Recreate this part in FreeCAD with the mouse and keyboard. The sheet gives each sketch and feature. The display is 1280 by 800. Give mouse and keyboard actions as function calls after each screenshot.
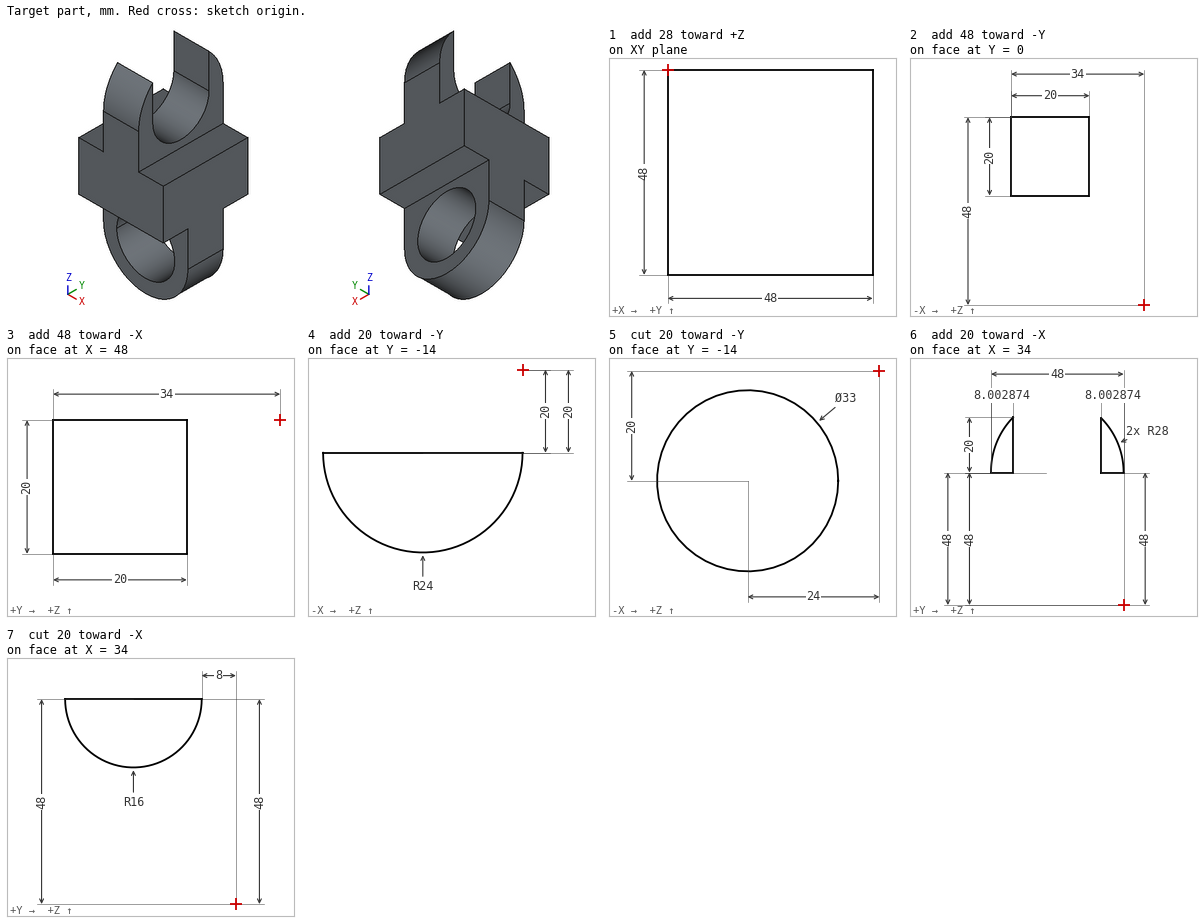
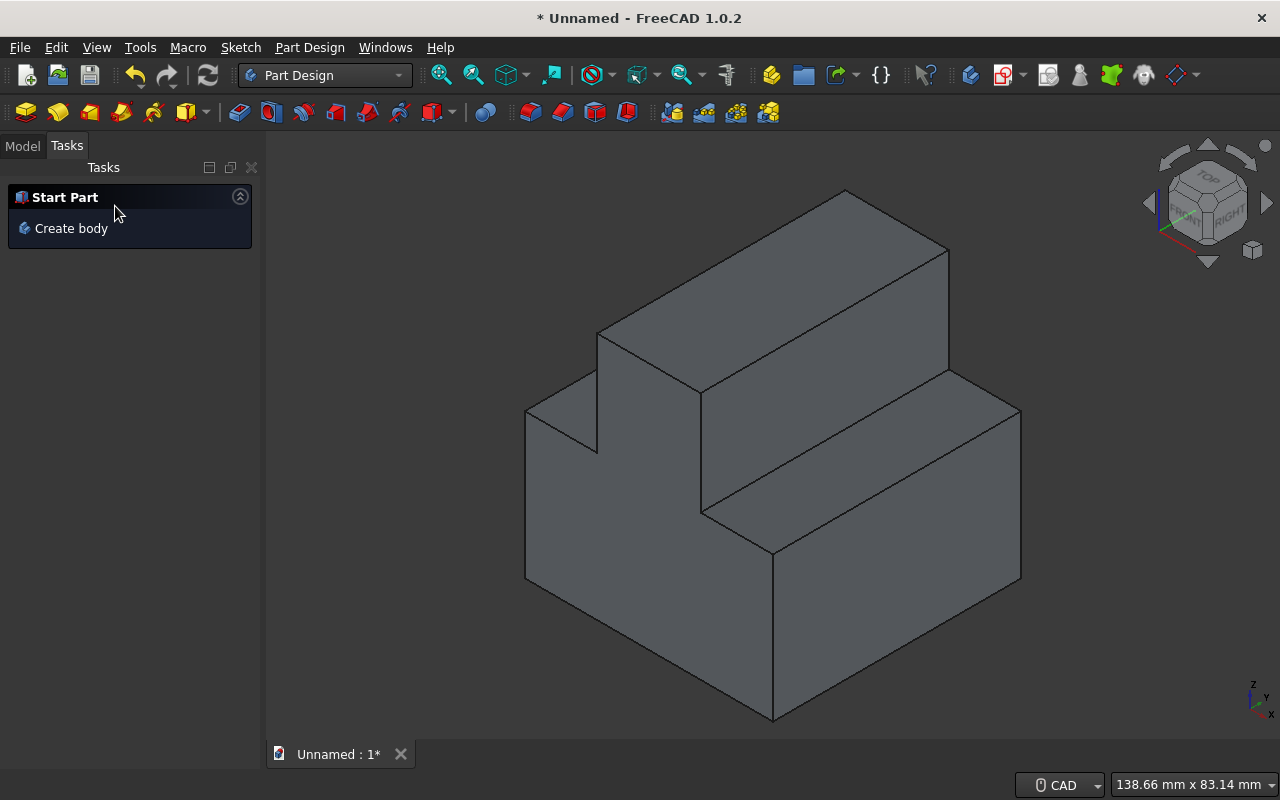
click(933, 545)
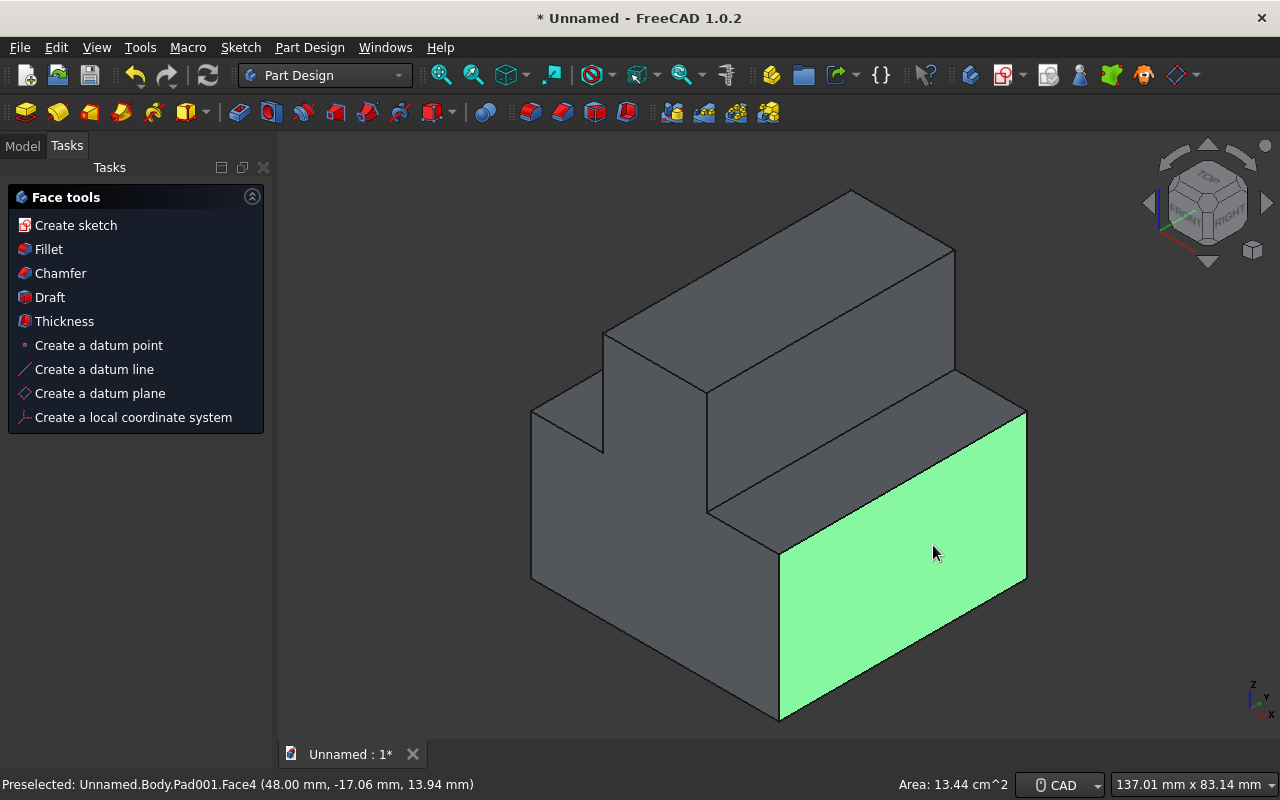
click(1004, 76)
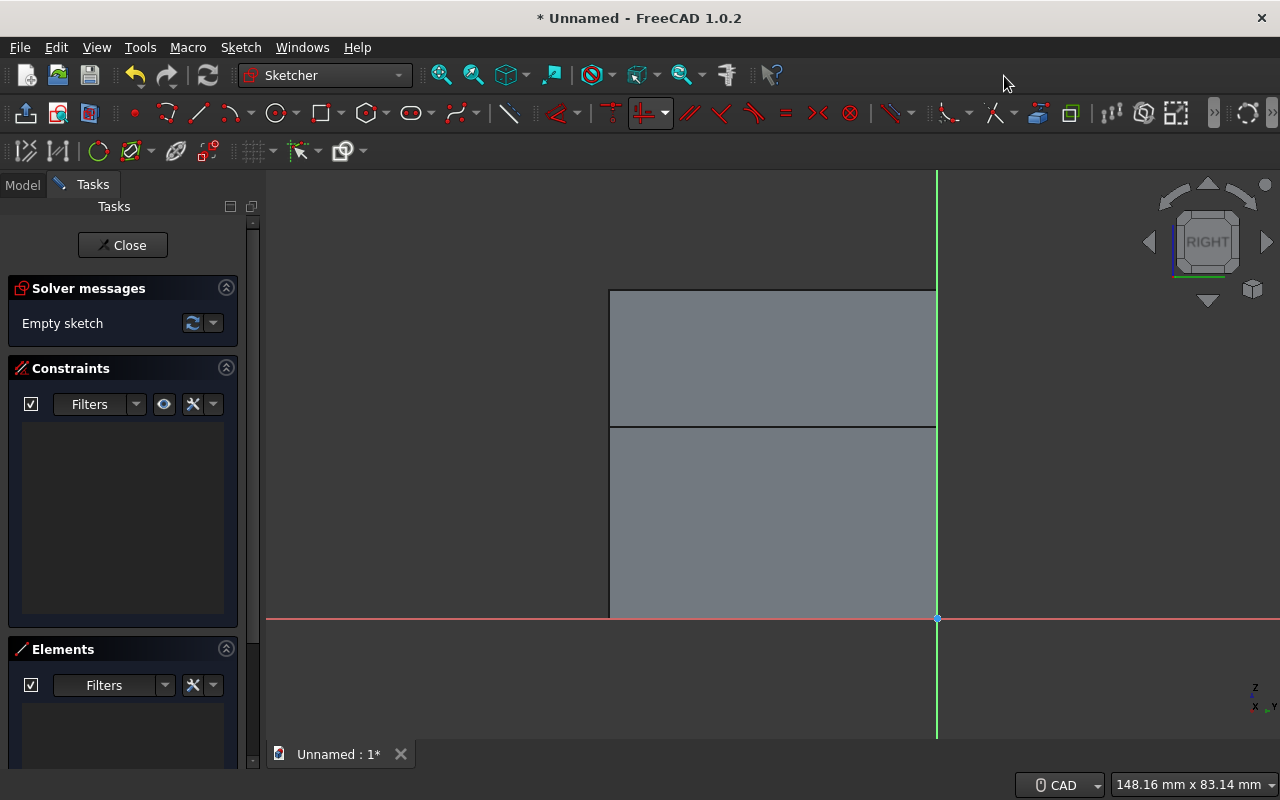
scroll(704, 454, down, 5)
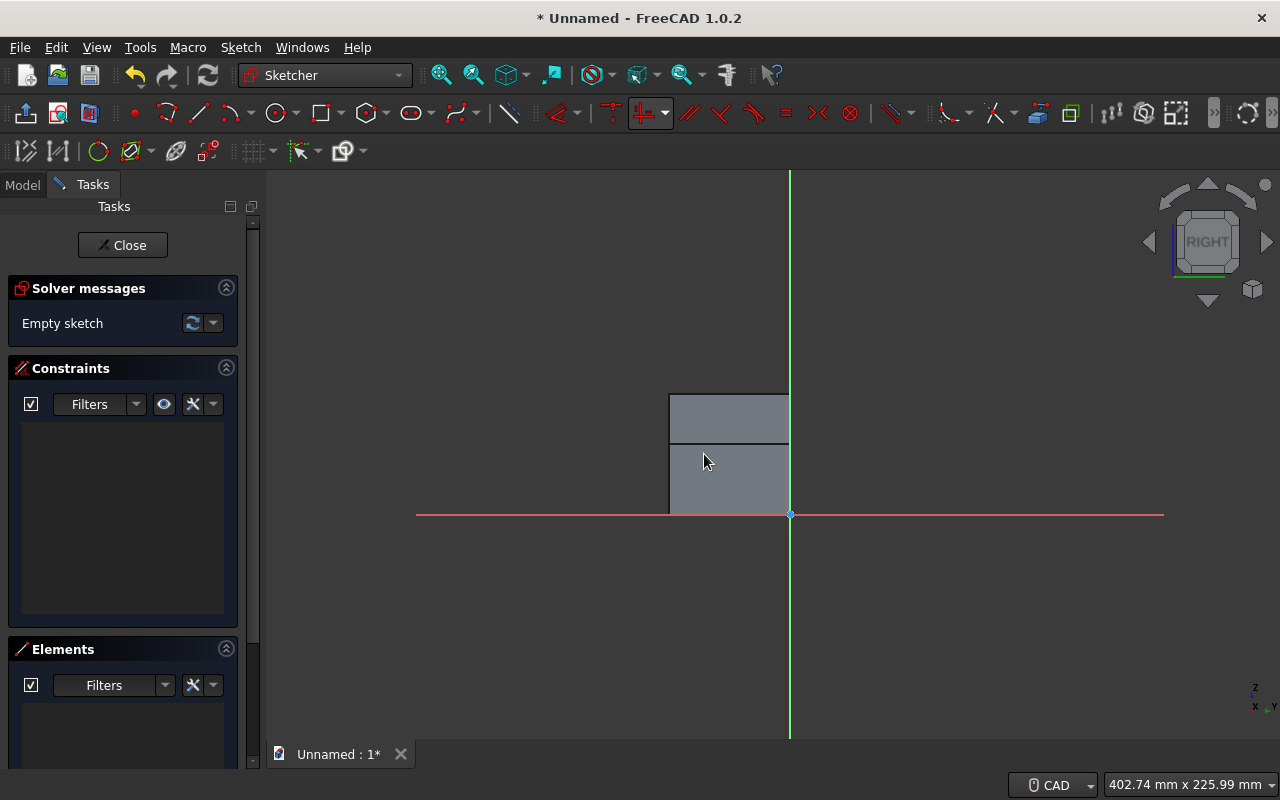
scroll(754, 554, up, 10)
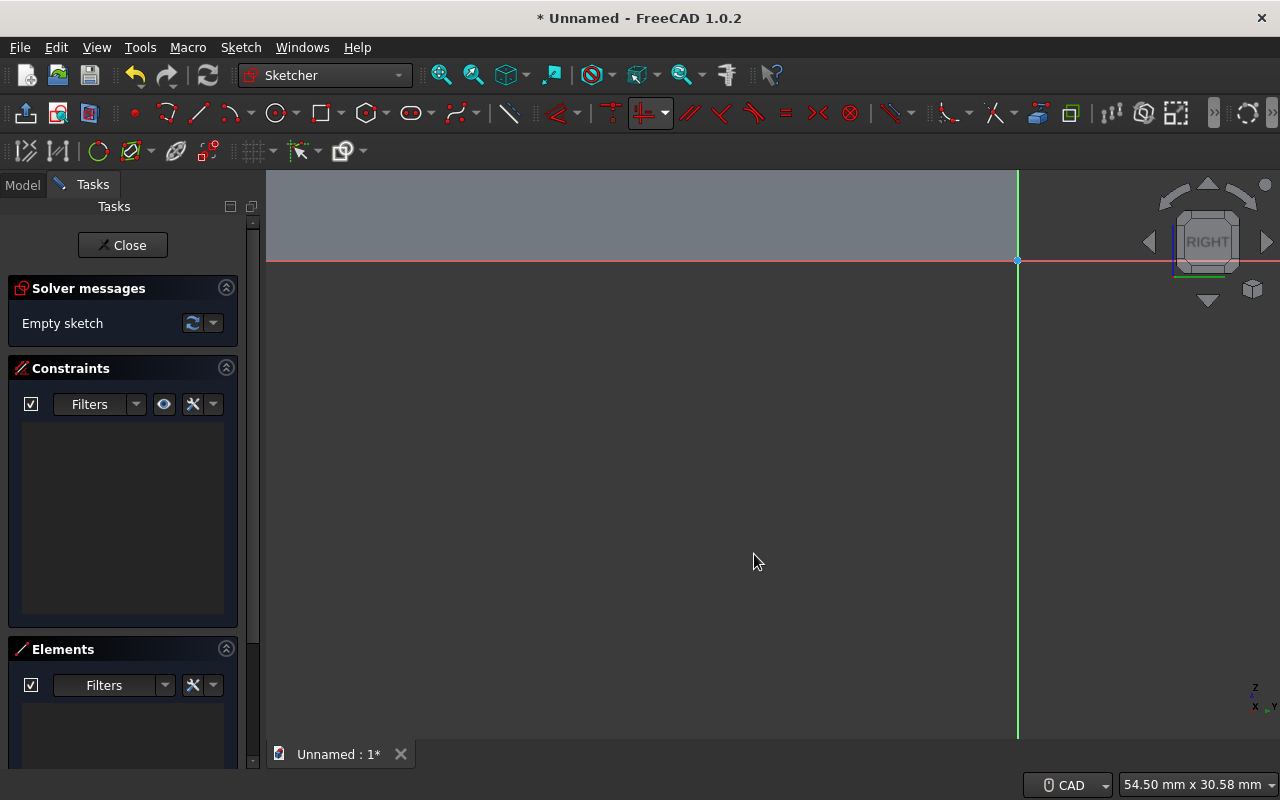
key(g)
key(r)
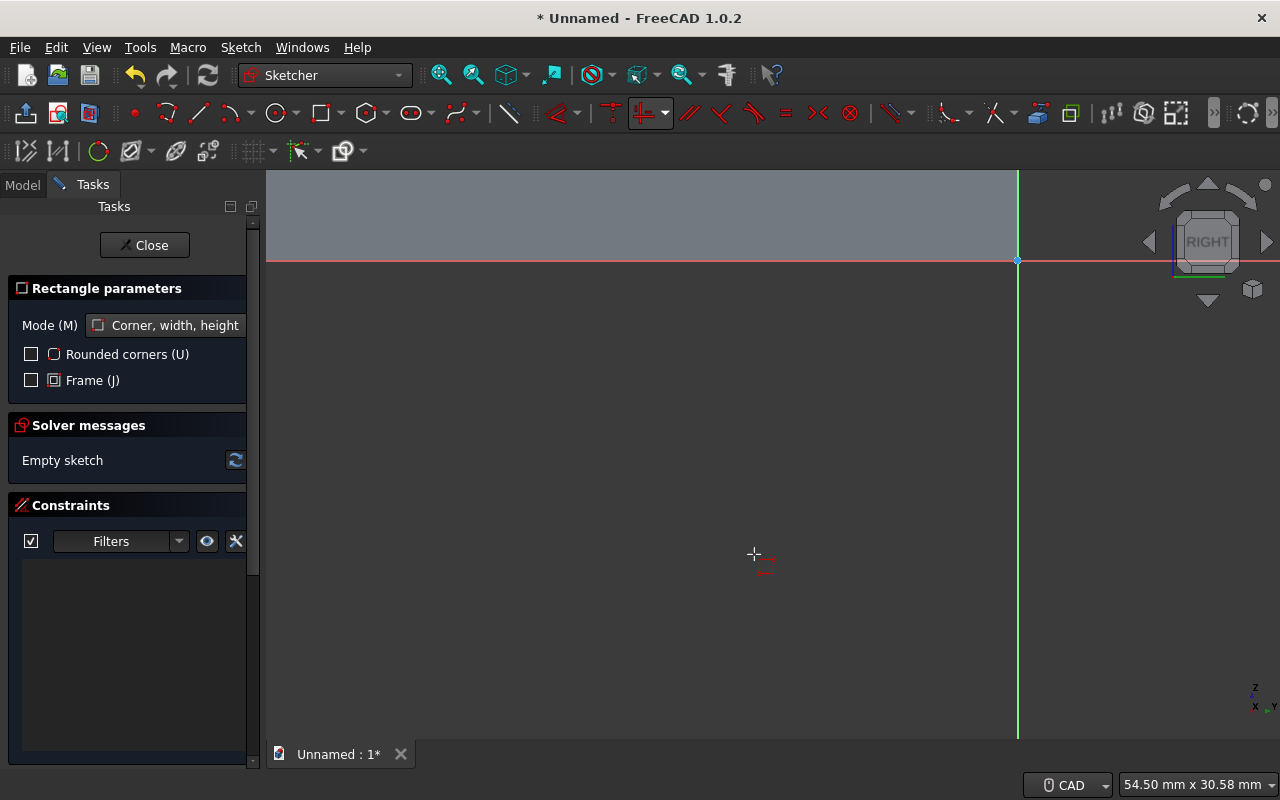
click(385, 261)
click(757, 633)
key(Escape)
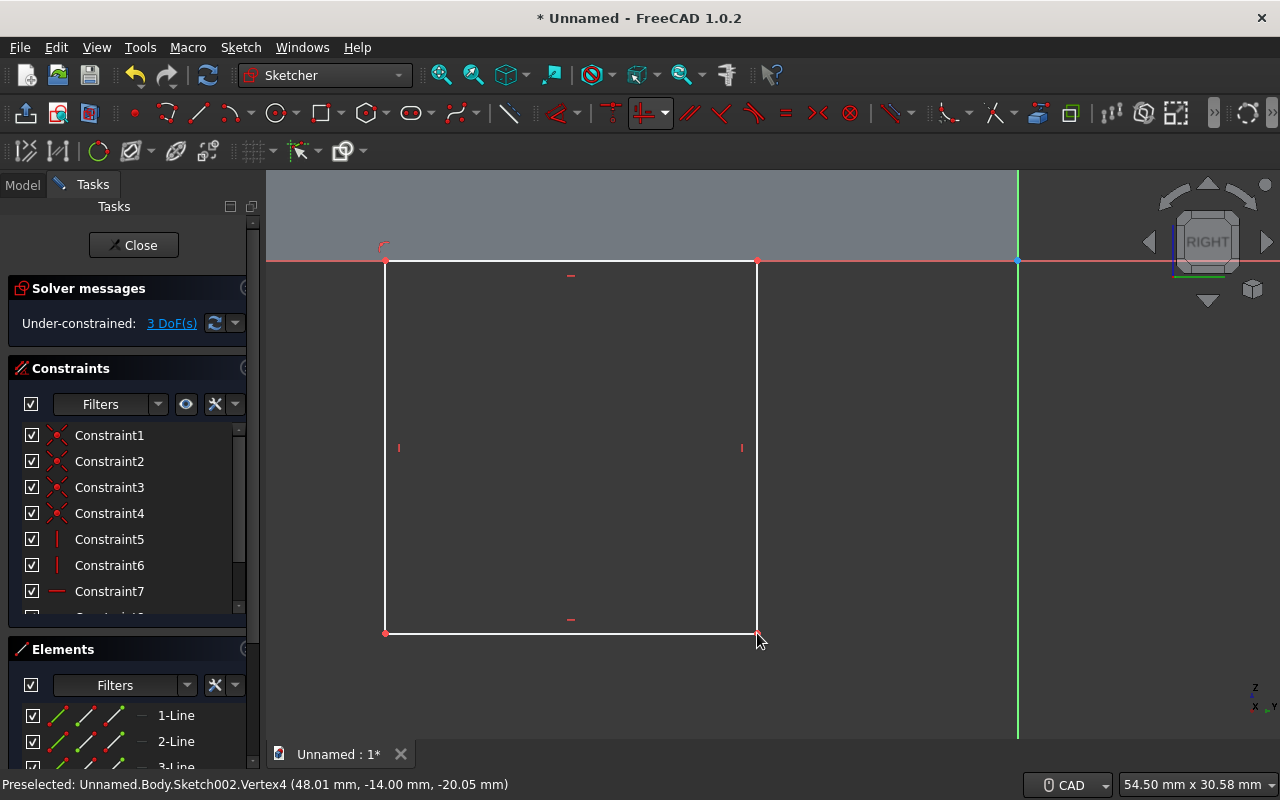
key(d)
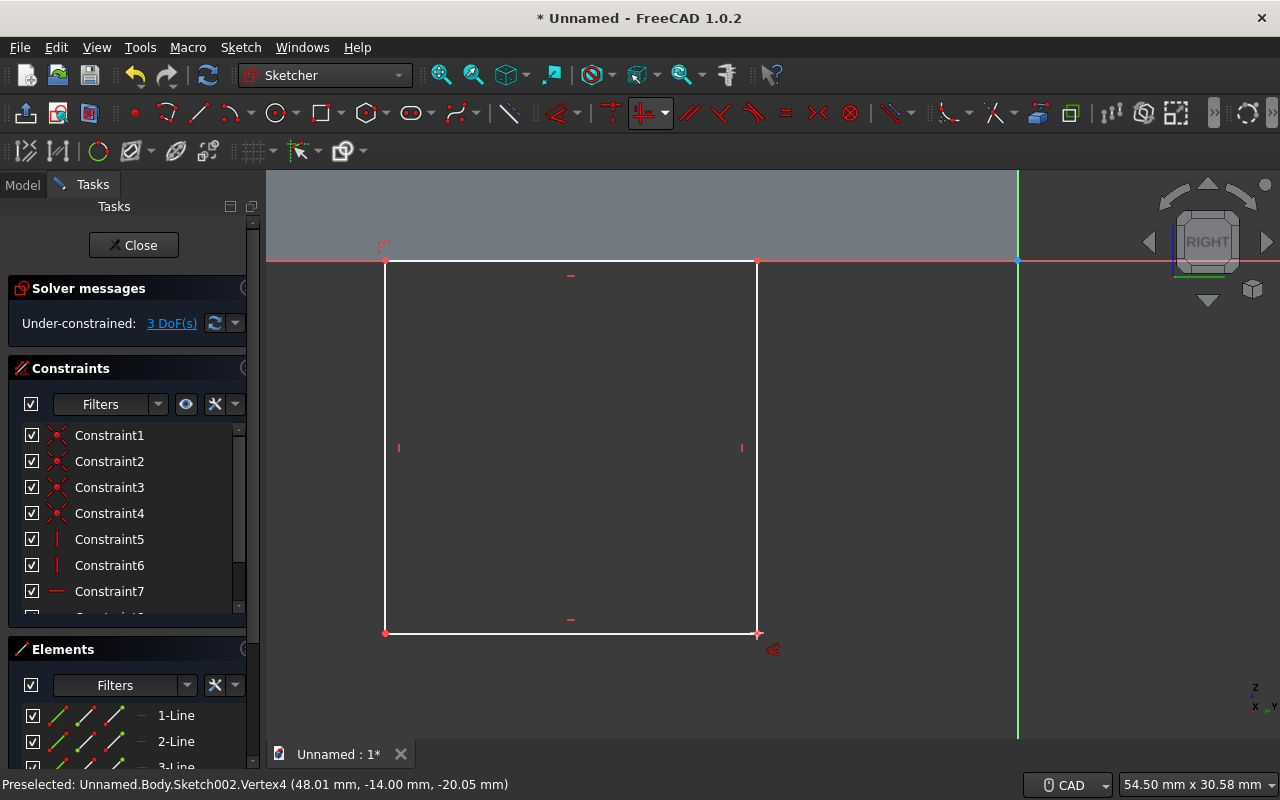
click(385, 373)
click(351, 447)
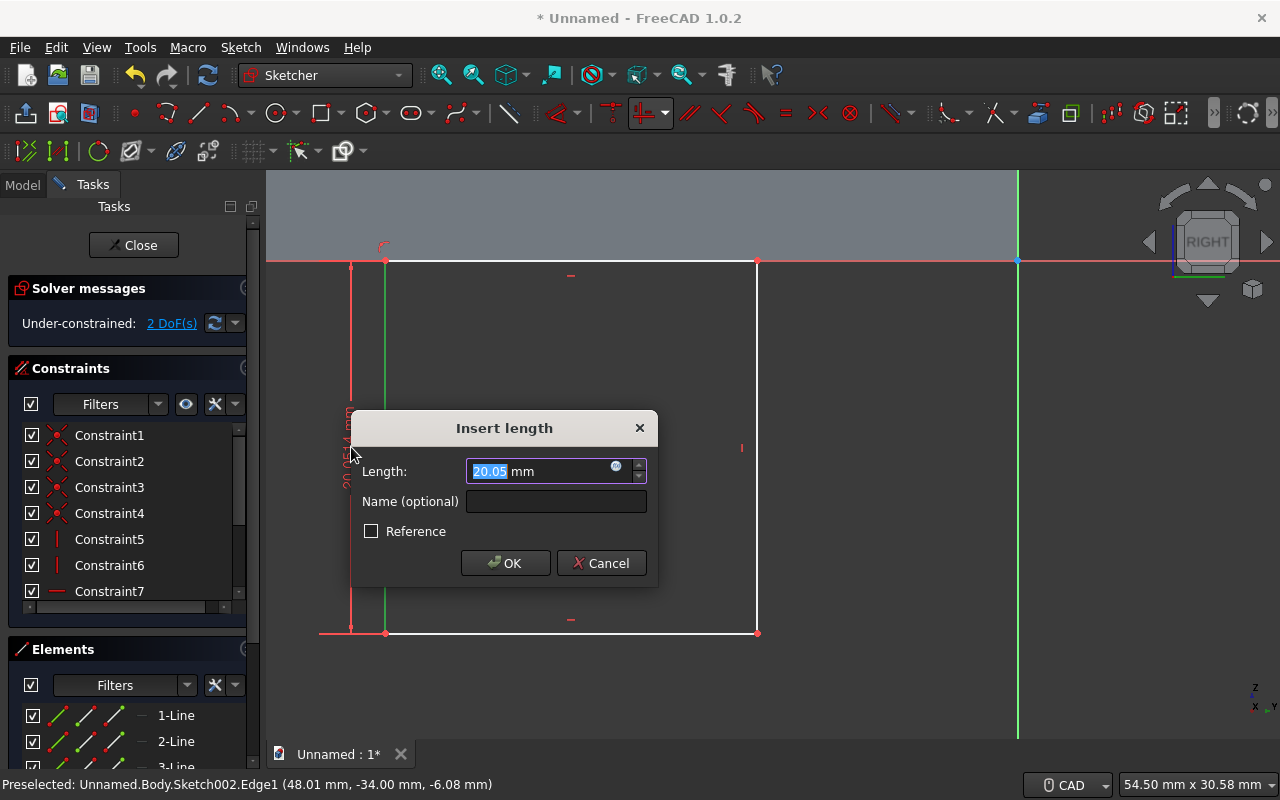
text(20)
key(Return)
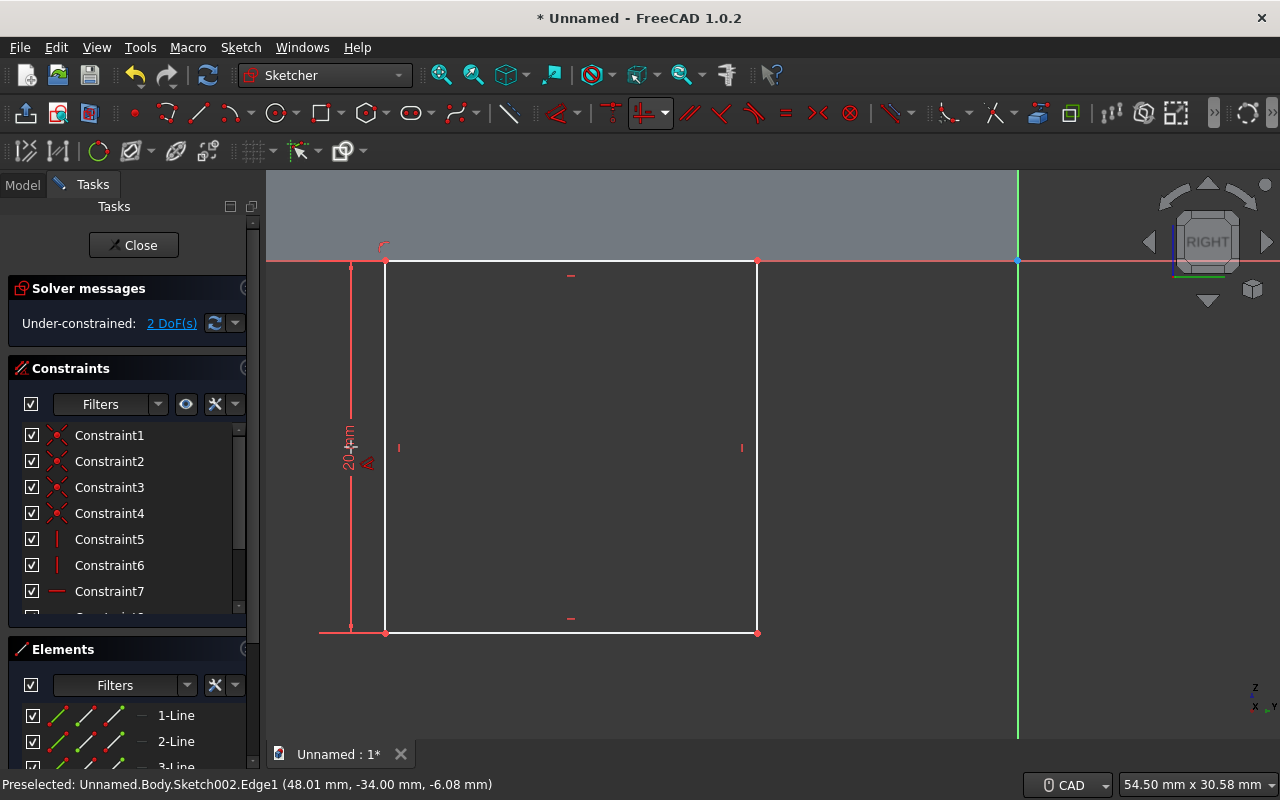
click(497, 633)
click(571, 667)